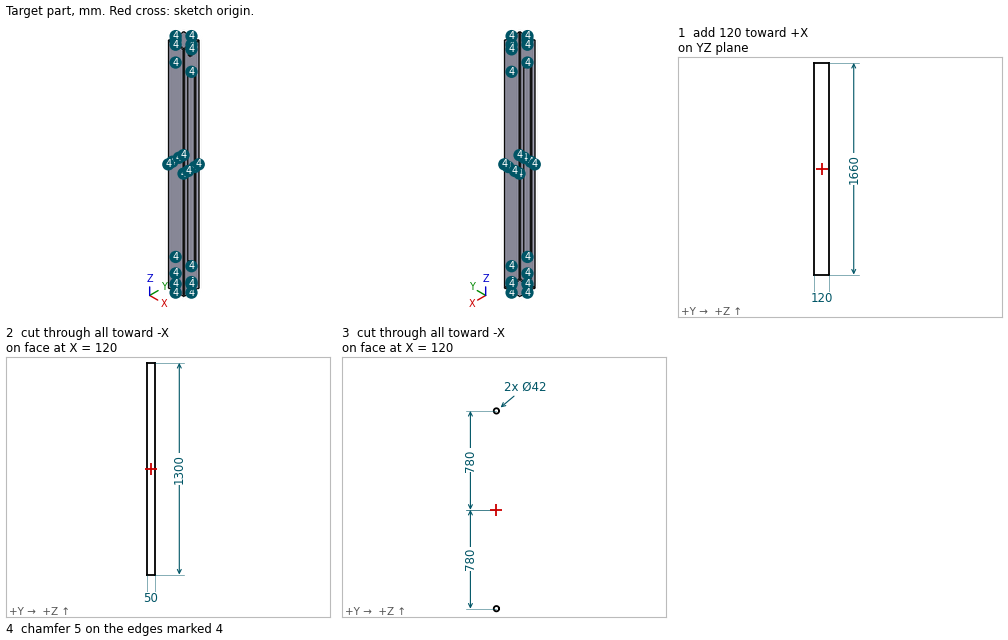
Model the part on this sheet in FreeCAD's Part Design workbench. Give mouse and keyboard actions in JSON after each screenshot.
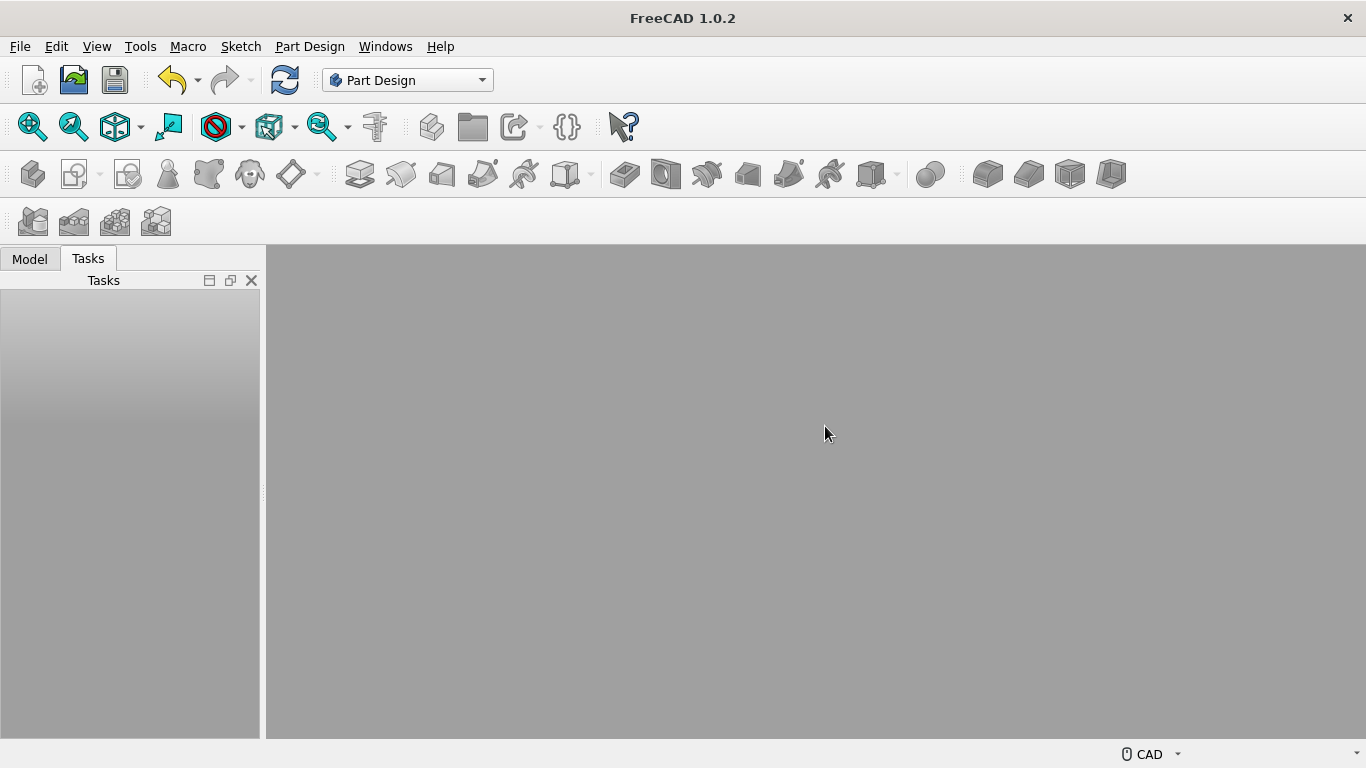
{"action": "left_click", "coordinate": [33, 80]}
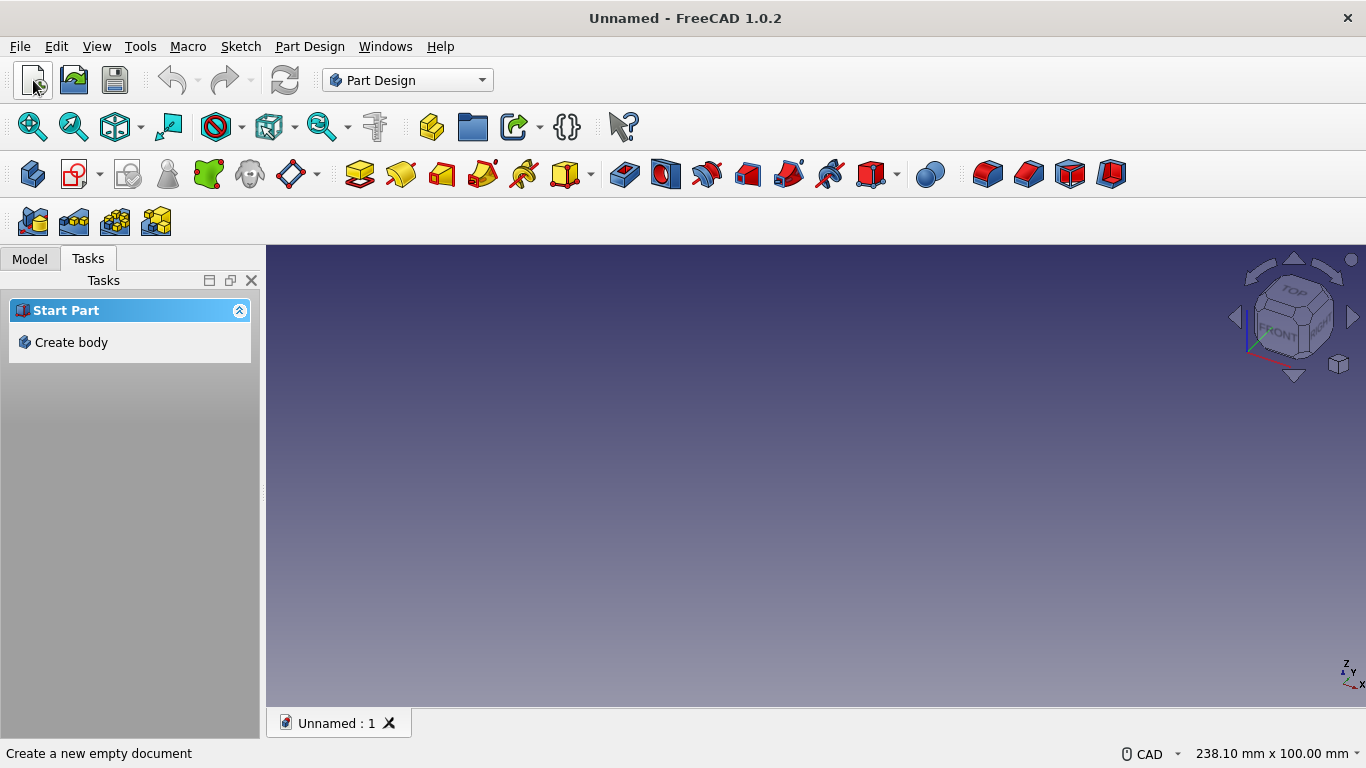
{"action": "left_click", "coordinate": [74, 174]}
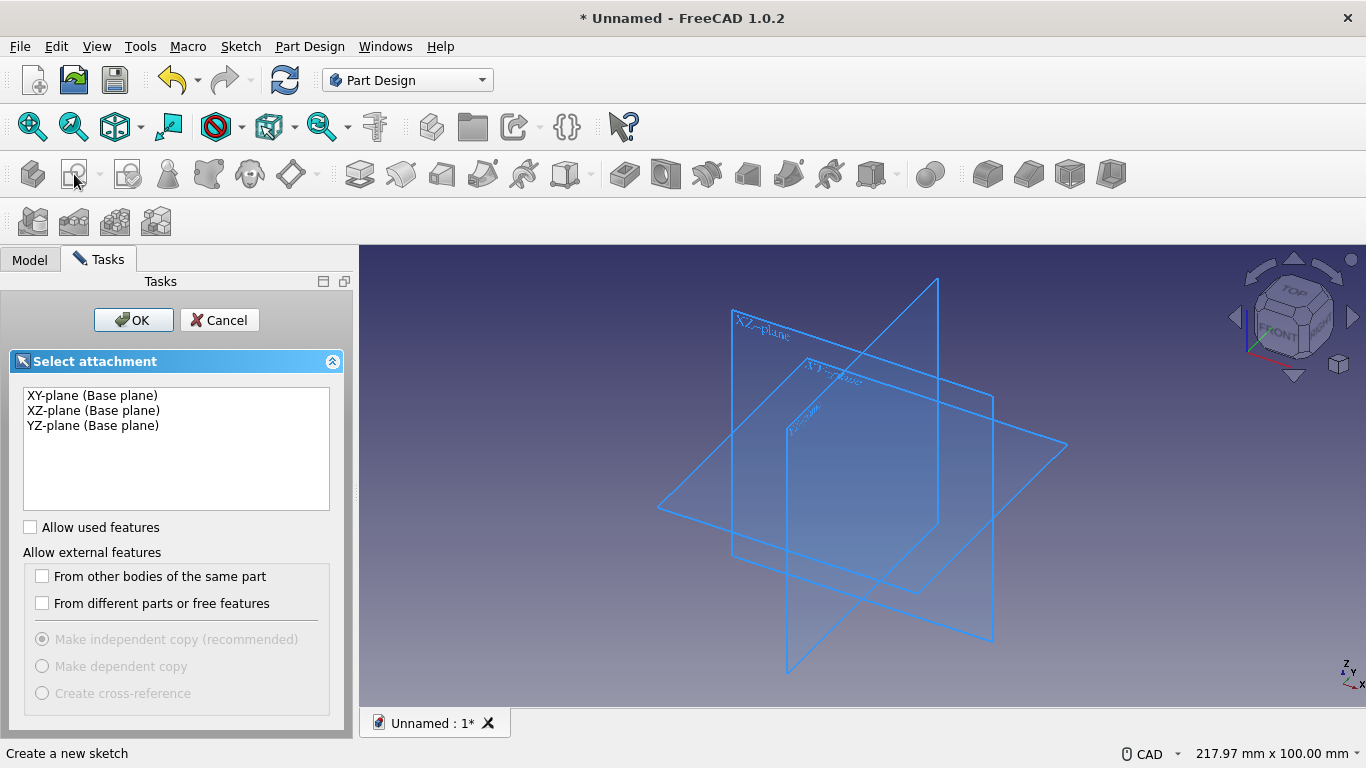
{"action": "left_click", "coordinate": [84, 426]}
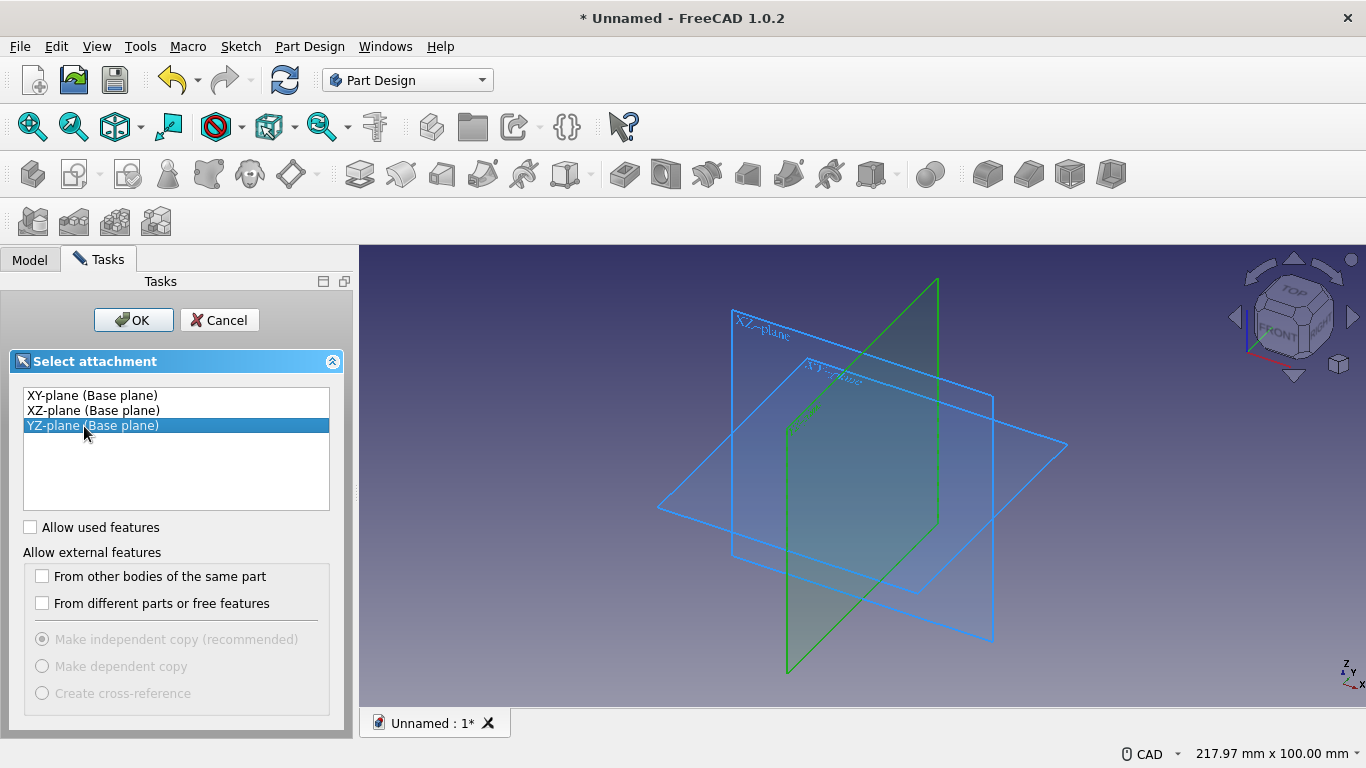
{"action": "left_click", "coordinate": [134, 320]}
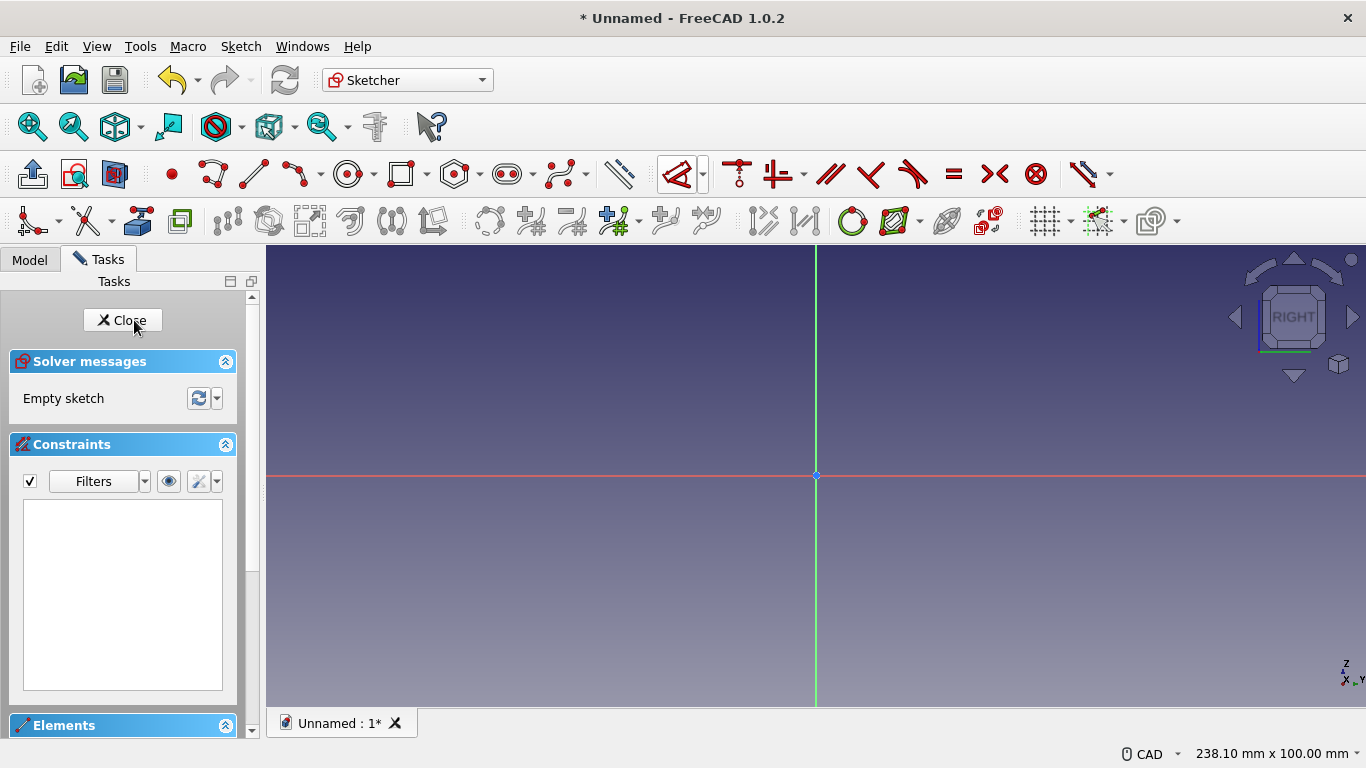
{"action": "scroll", "coordinate": [745, 476], "scroll_direction": "down", "scroll_amount": 16}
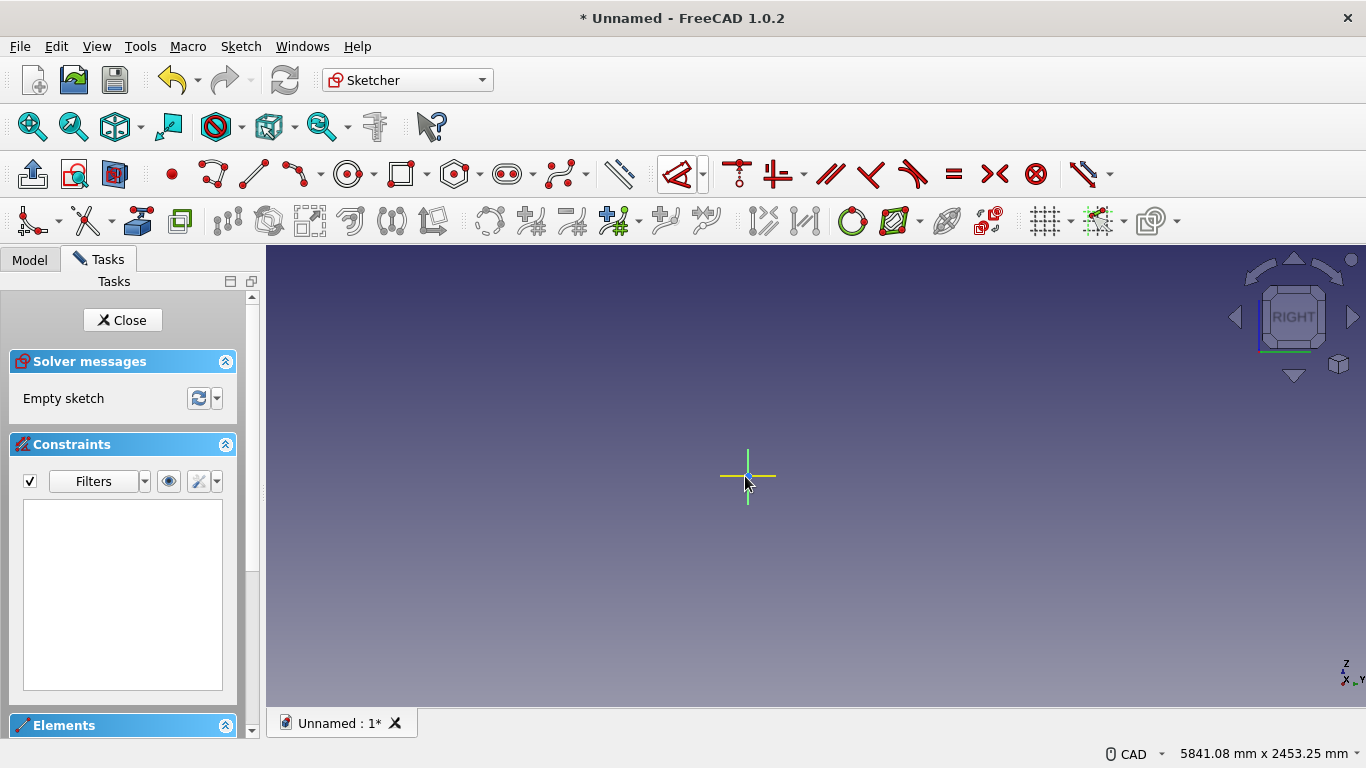
{"action": "key", "text": "g v"}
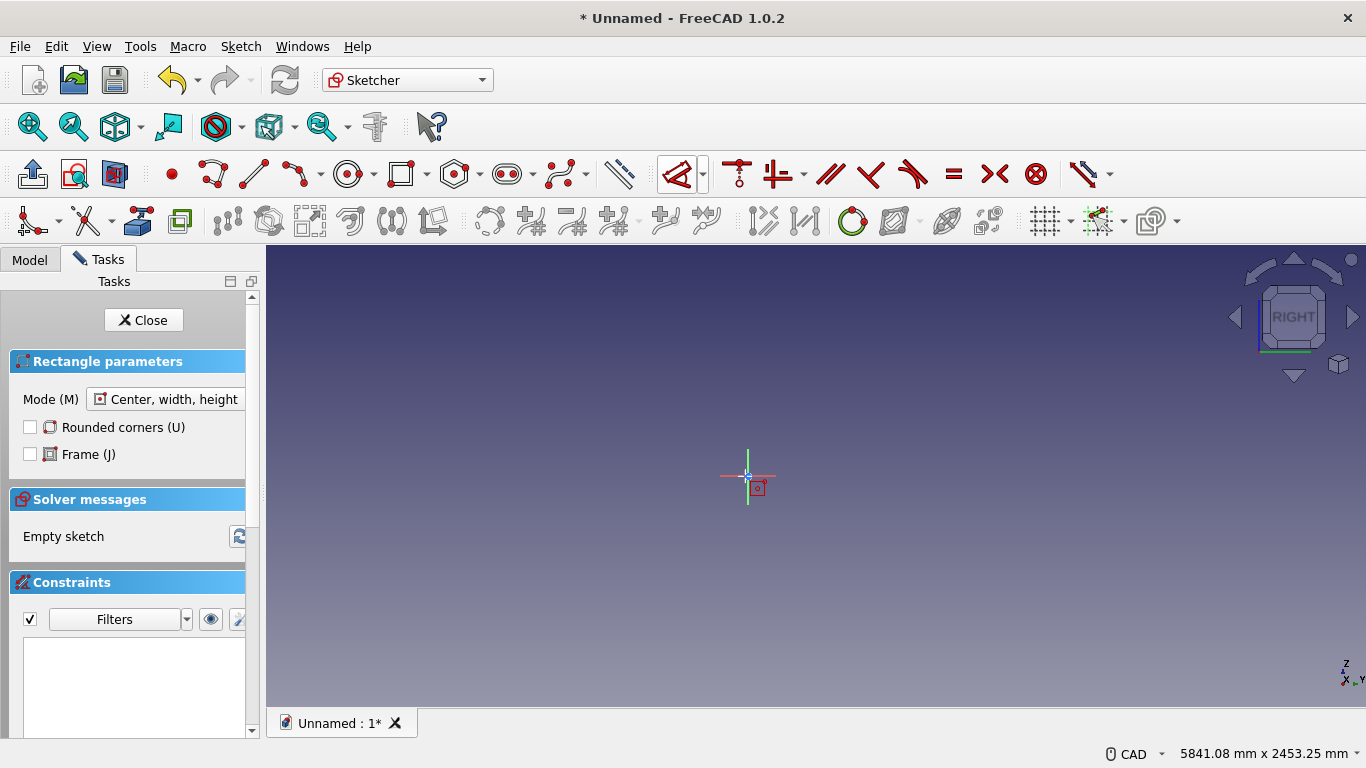
{"action": "scroll", "coordinate": [748, 476], "scroll_direction": "up", "scroll_amount": 2}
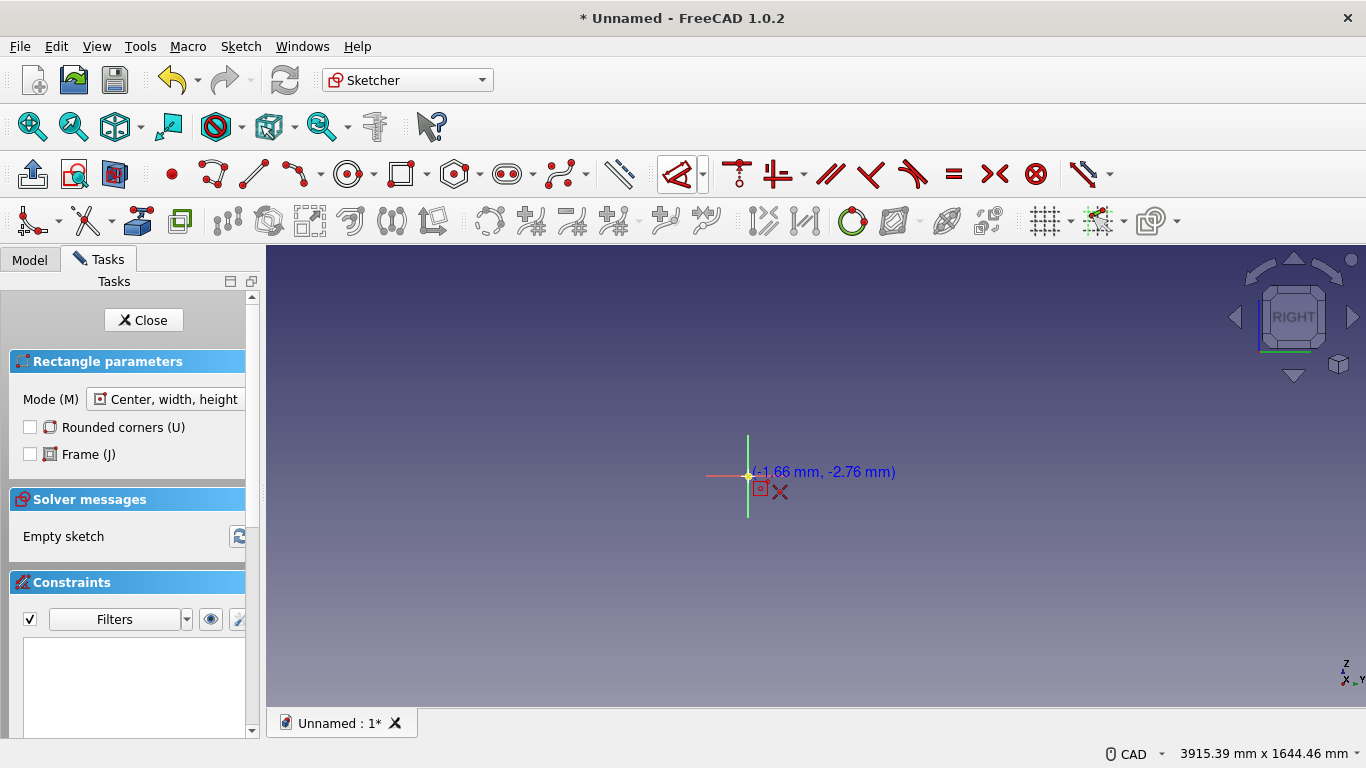
{"action": "left_click", "coordinate": [748, 476]}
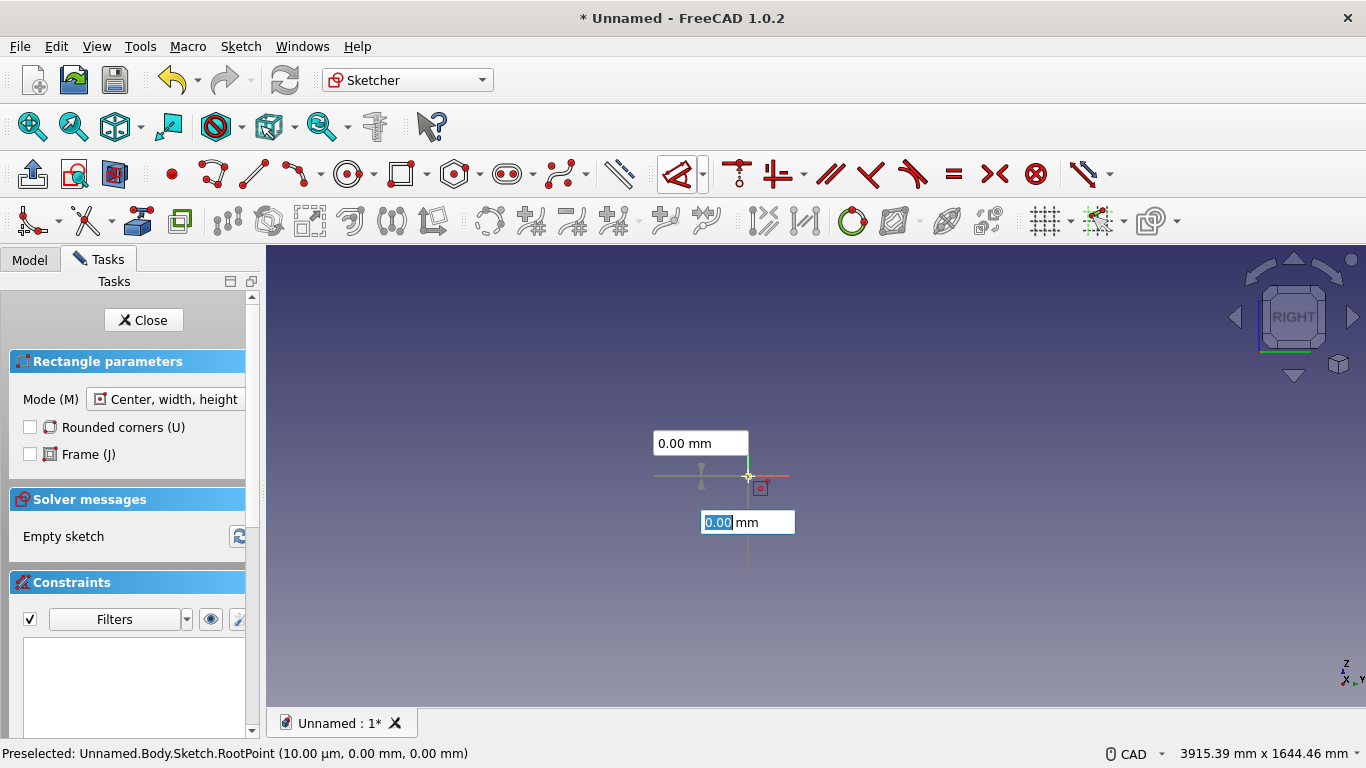
{"action": "scroll", "coordinate": [746, 475], "scroll_direction": "down", "scroll_amount": 2}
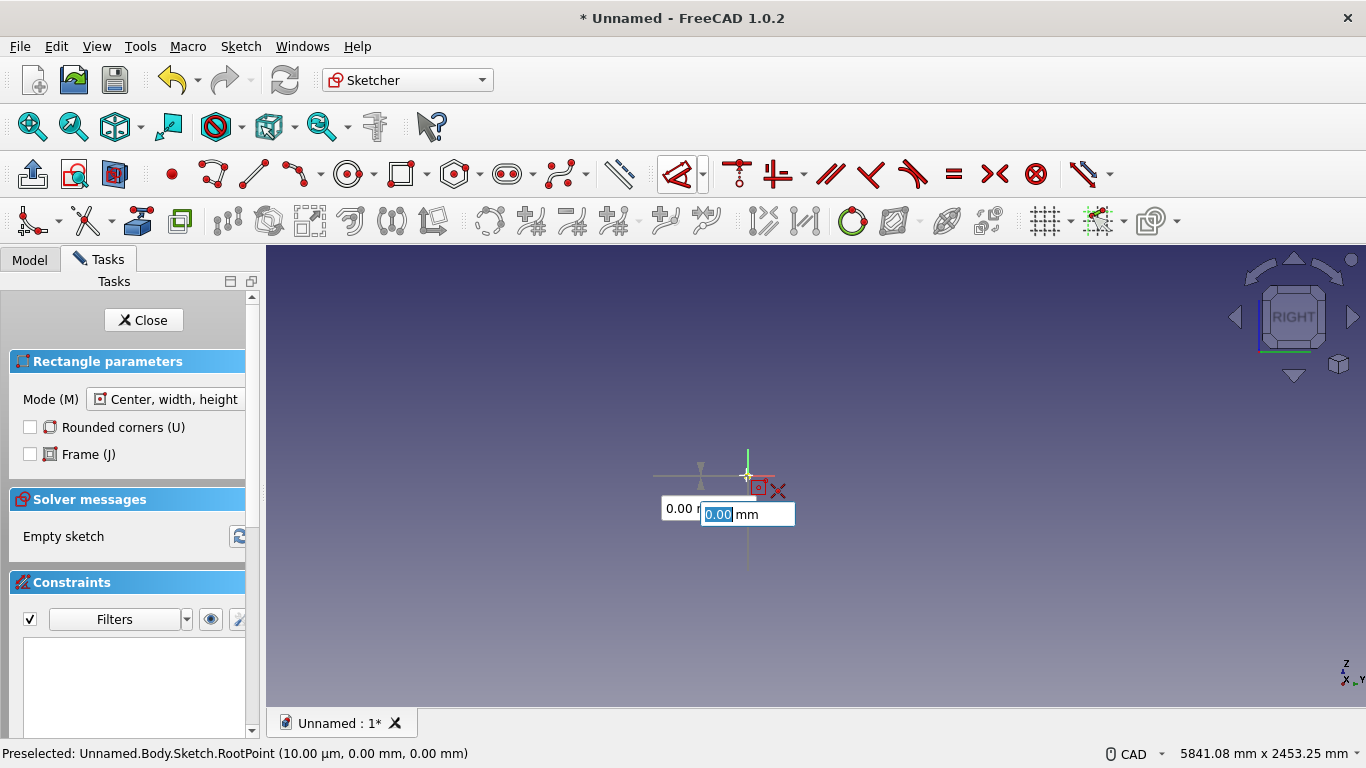
{"action": "scroll", "coordinate": [759, 320], "scroll_direction": "up", "scroll_amount": 2}